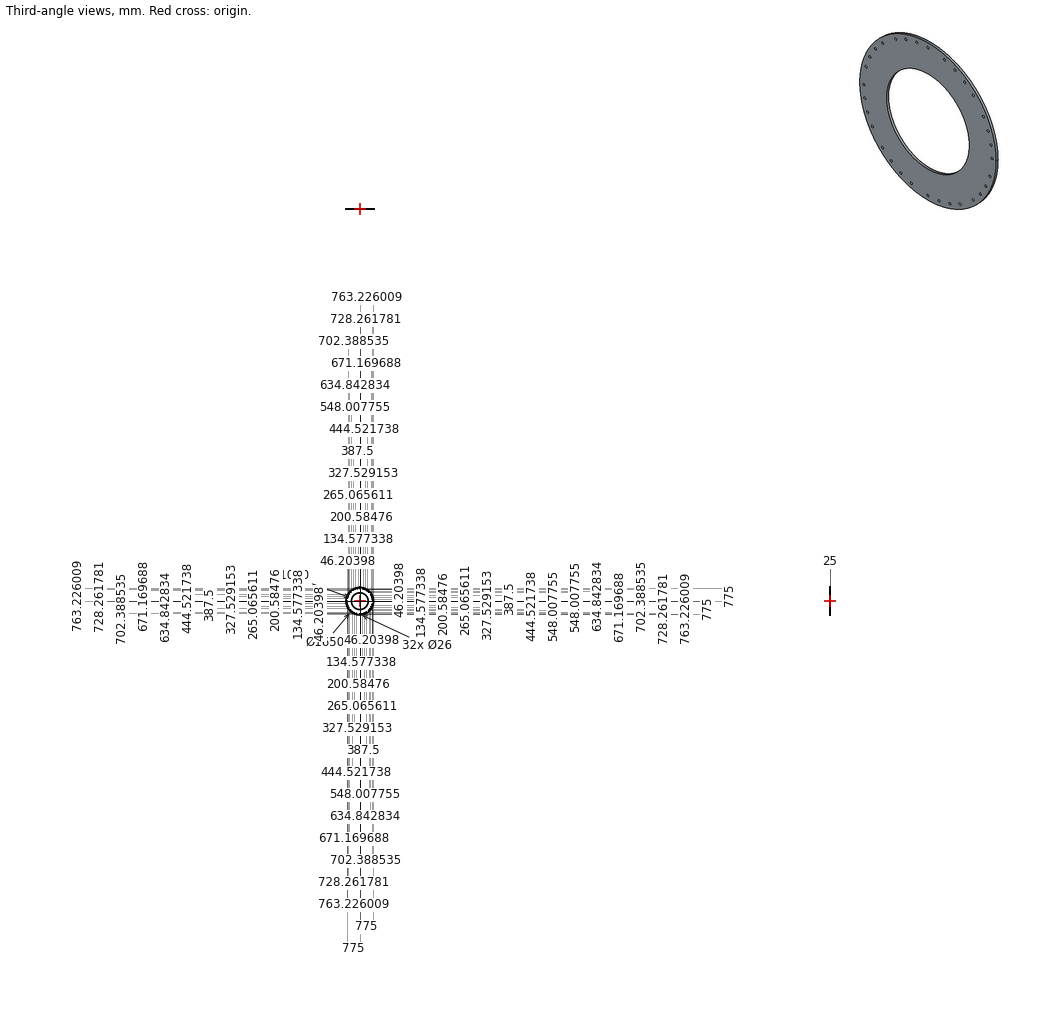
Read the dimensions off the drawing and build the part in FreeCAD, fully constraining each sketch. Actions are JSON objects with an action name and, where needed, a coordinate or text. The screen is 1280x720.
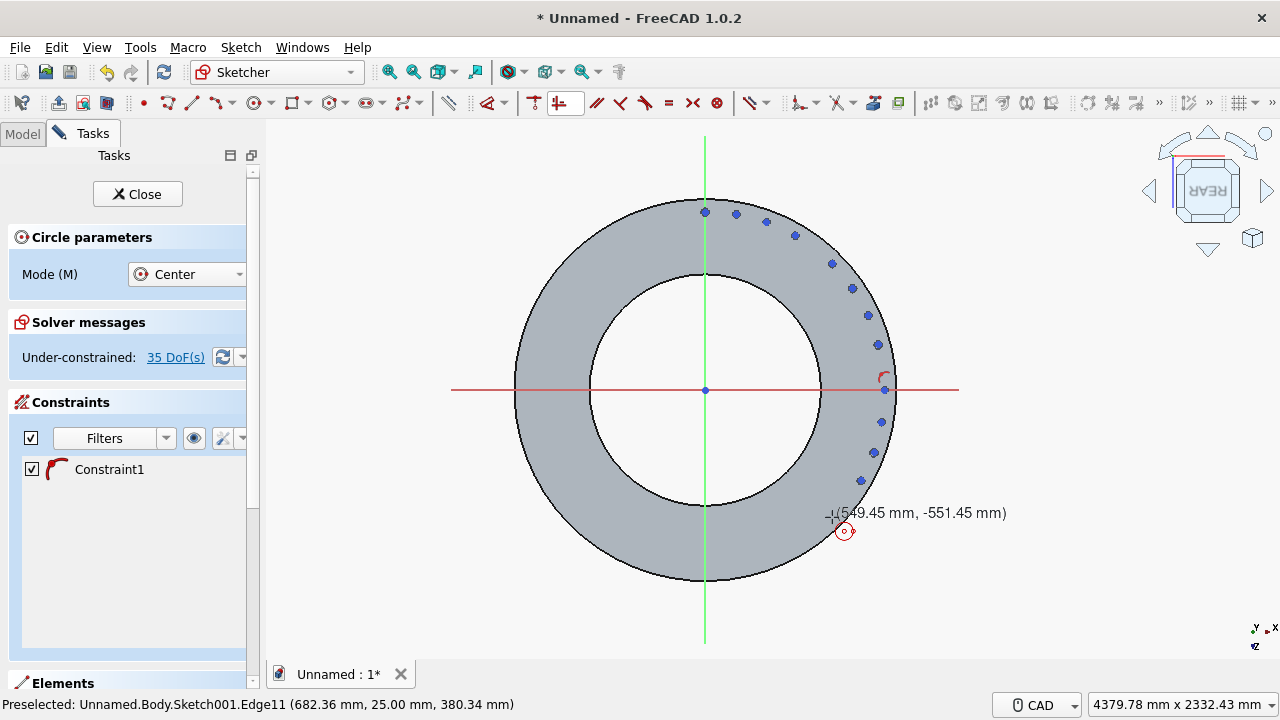
{"action": "left_click", "coordinate": [832, 517]}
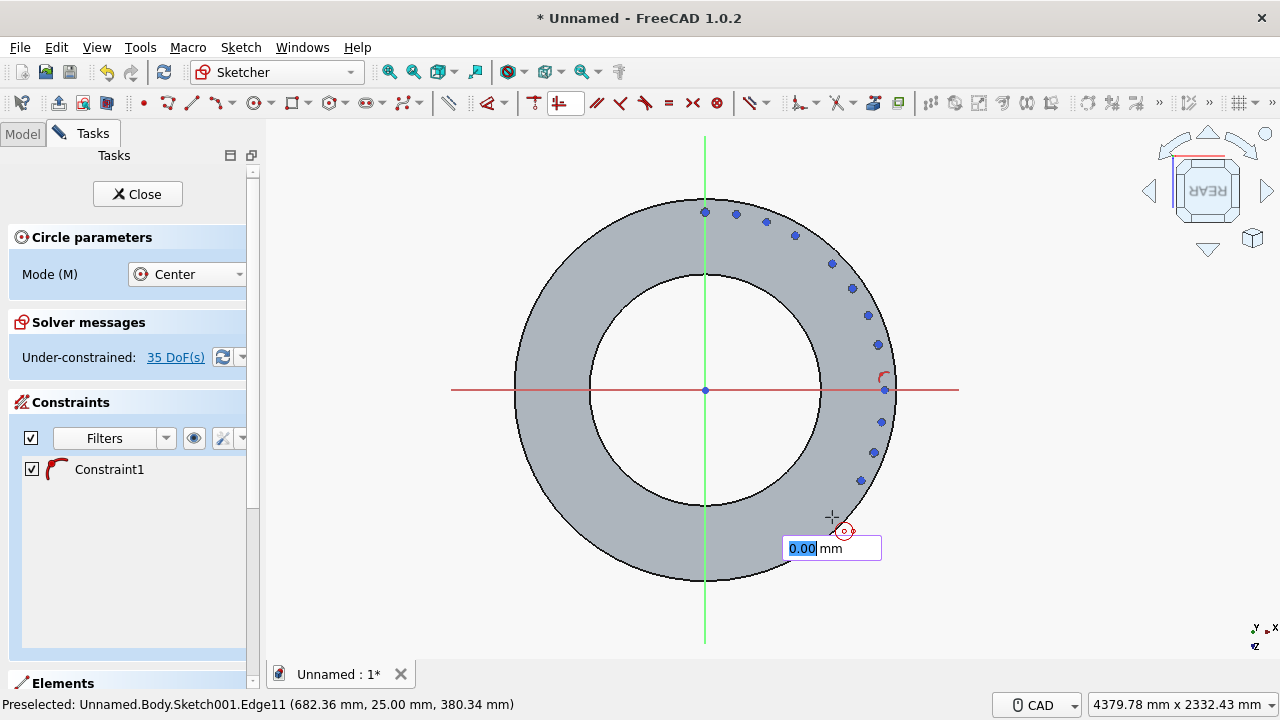
{"action": "scroll", "coordinate": [834, 515], "scroll_direction": "up", "scroll_amount": 9}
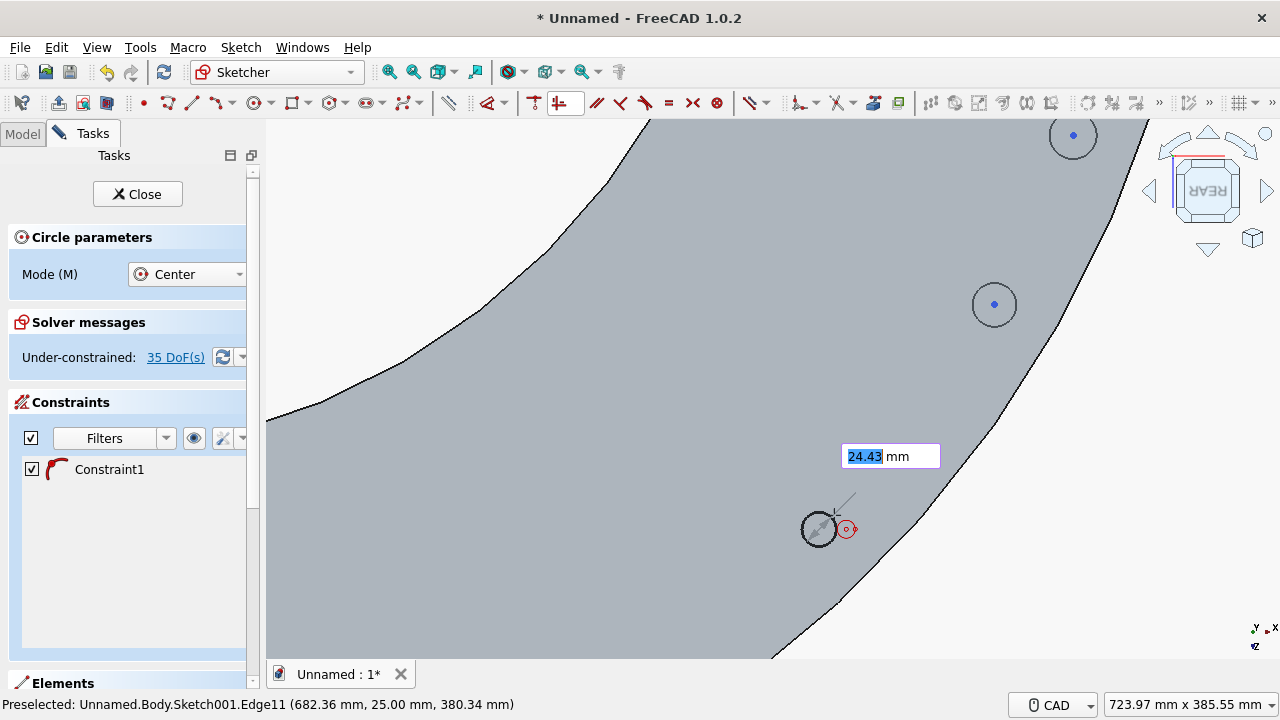
{"action": "left_click", "coordinate": [833, 510]}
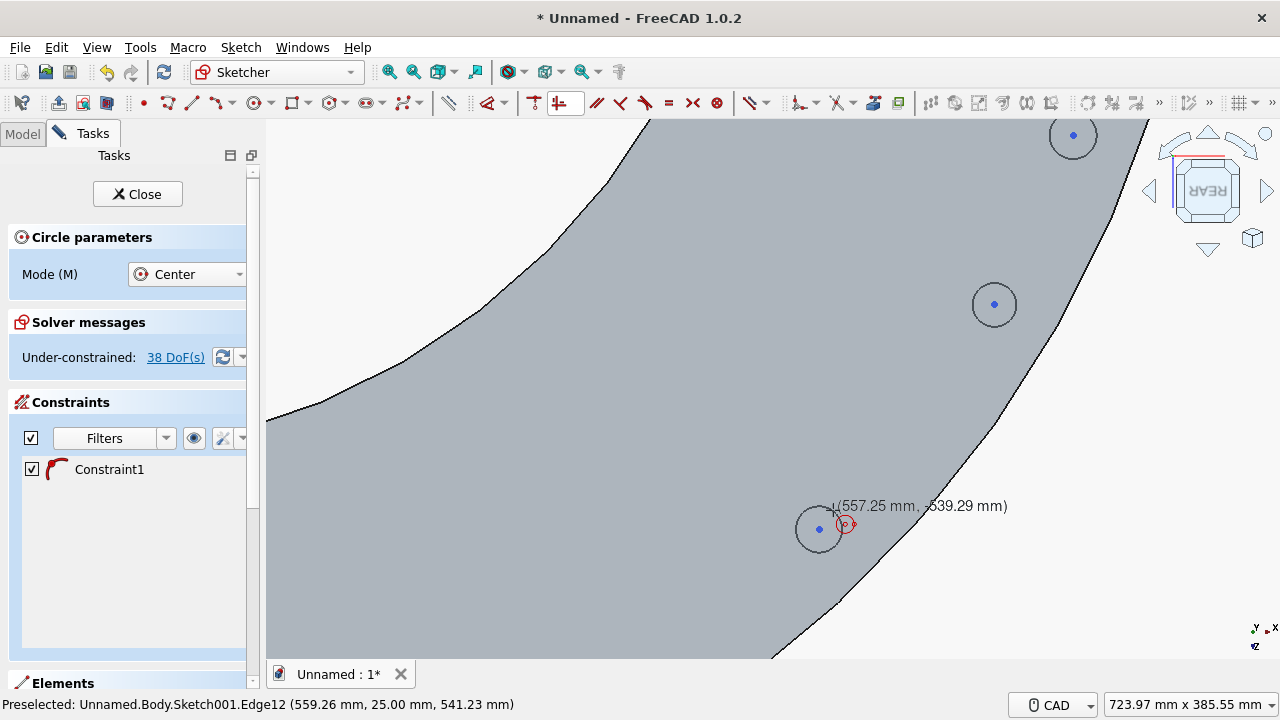
{"action": "scroll", "coordinate": [834, 514], "scroll_direction": "down", "scroll_amount": 9}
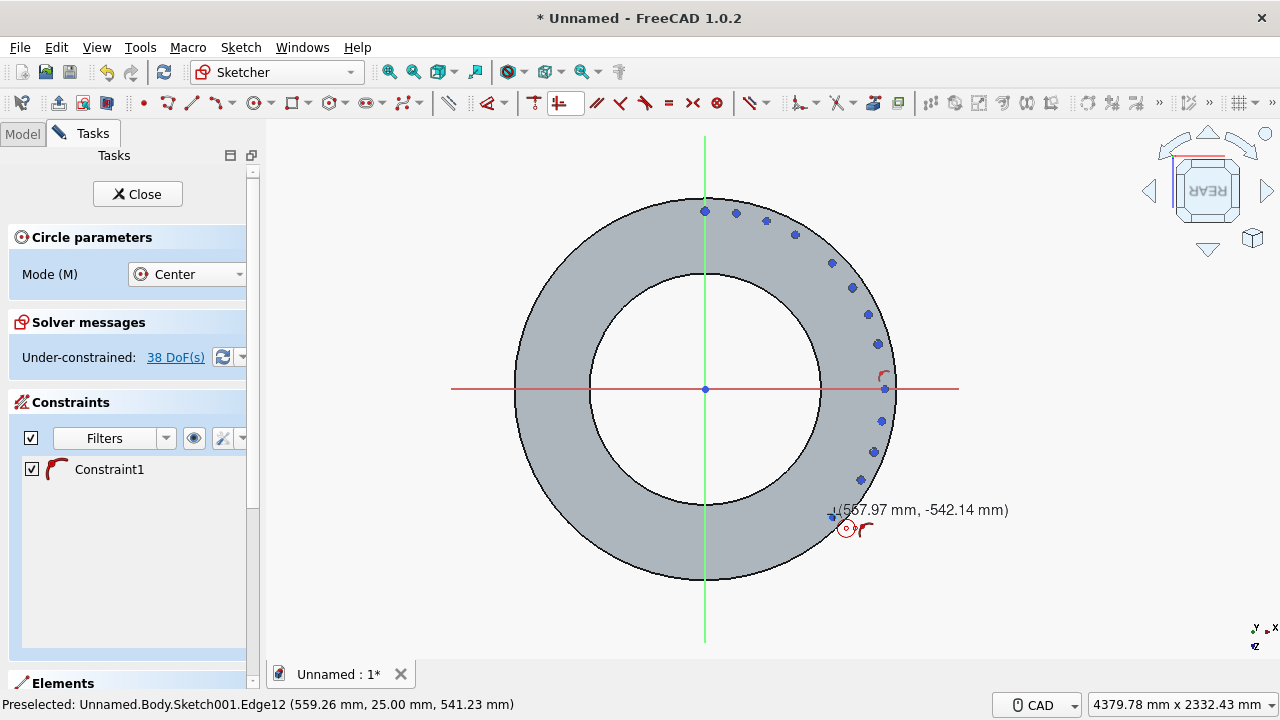
{"action": "scroll", "coordinate": [808, 536], "scroll_direction": "up", "scroll_amount": 11}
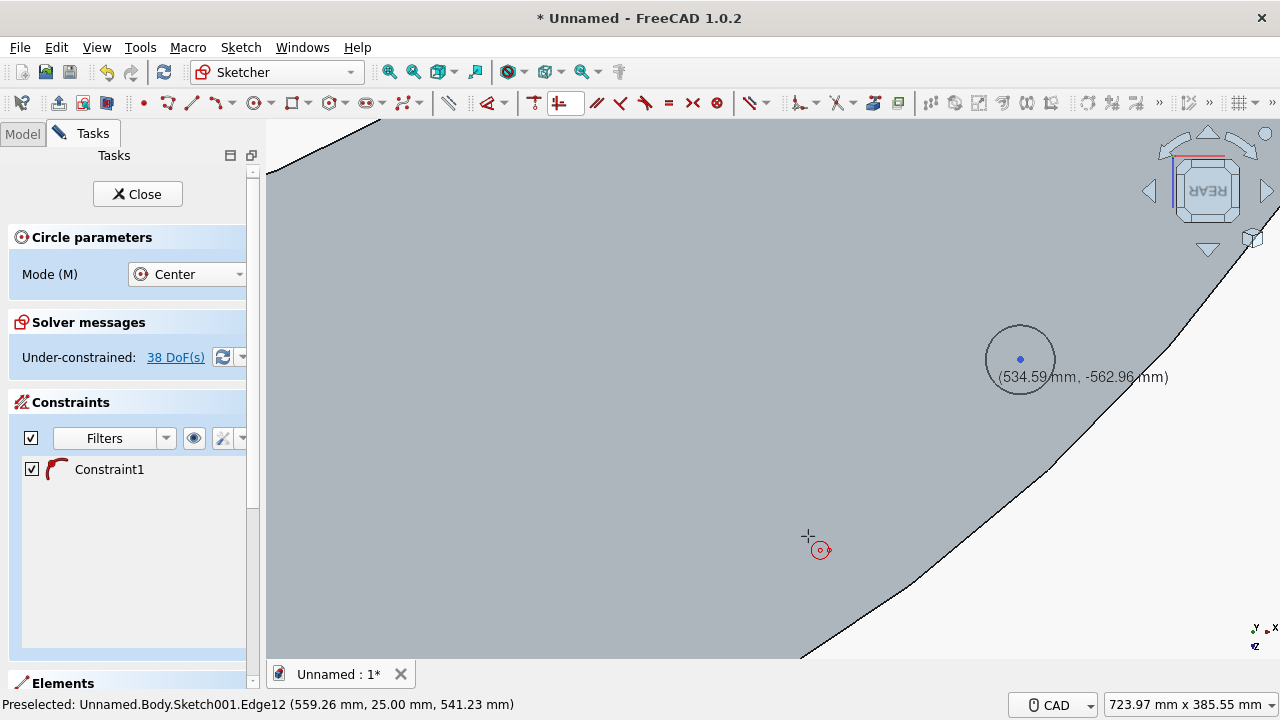
{"action": "scroll", "coordinate": [808, 536], "scroll_direction": "down", "scroll_amount": 11}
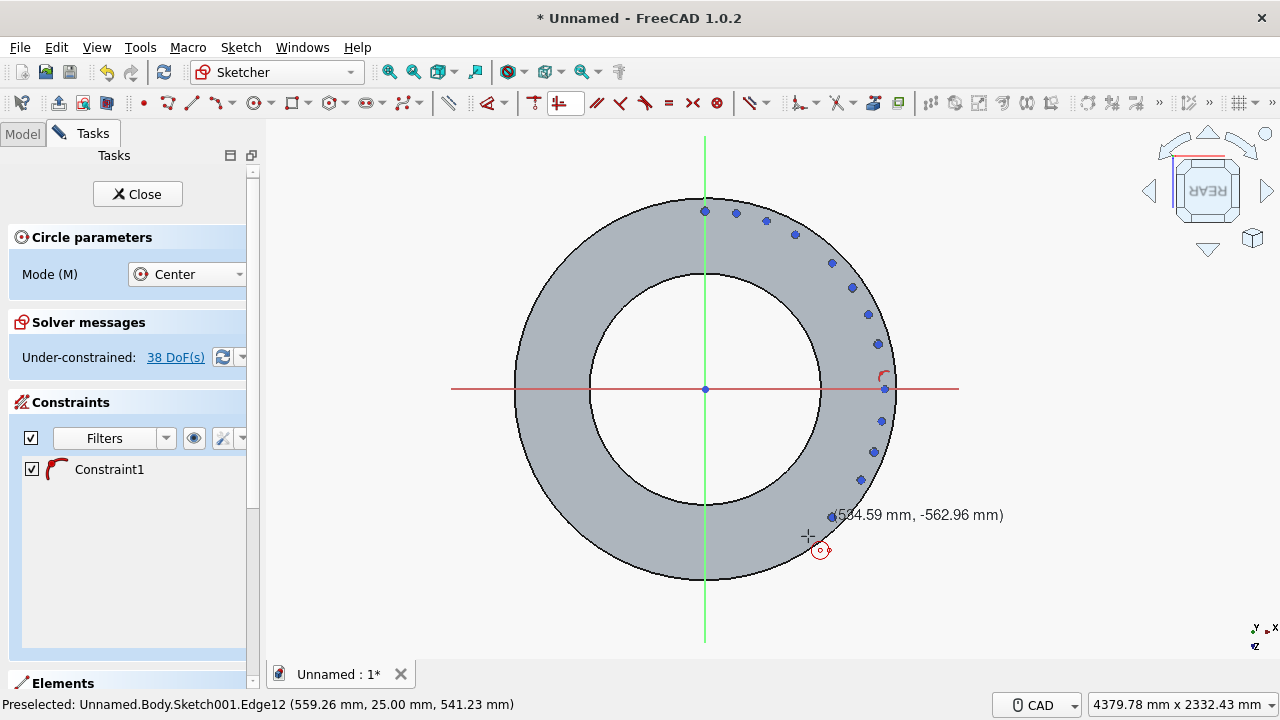
{"action": "left_click", "coordinate": [808, 536]}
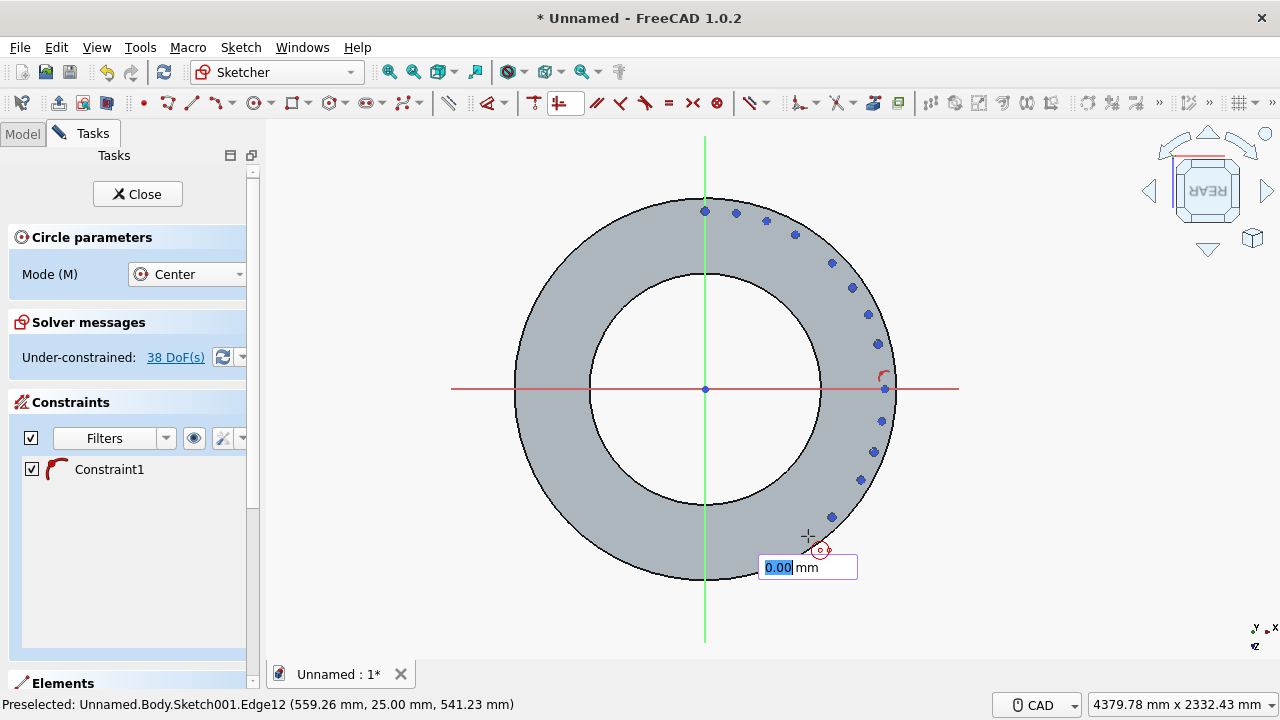
{"action": "scroll", "coordinate": [810, 534], "scroll_direction": "up", "scroll_amount": 9}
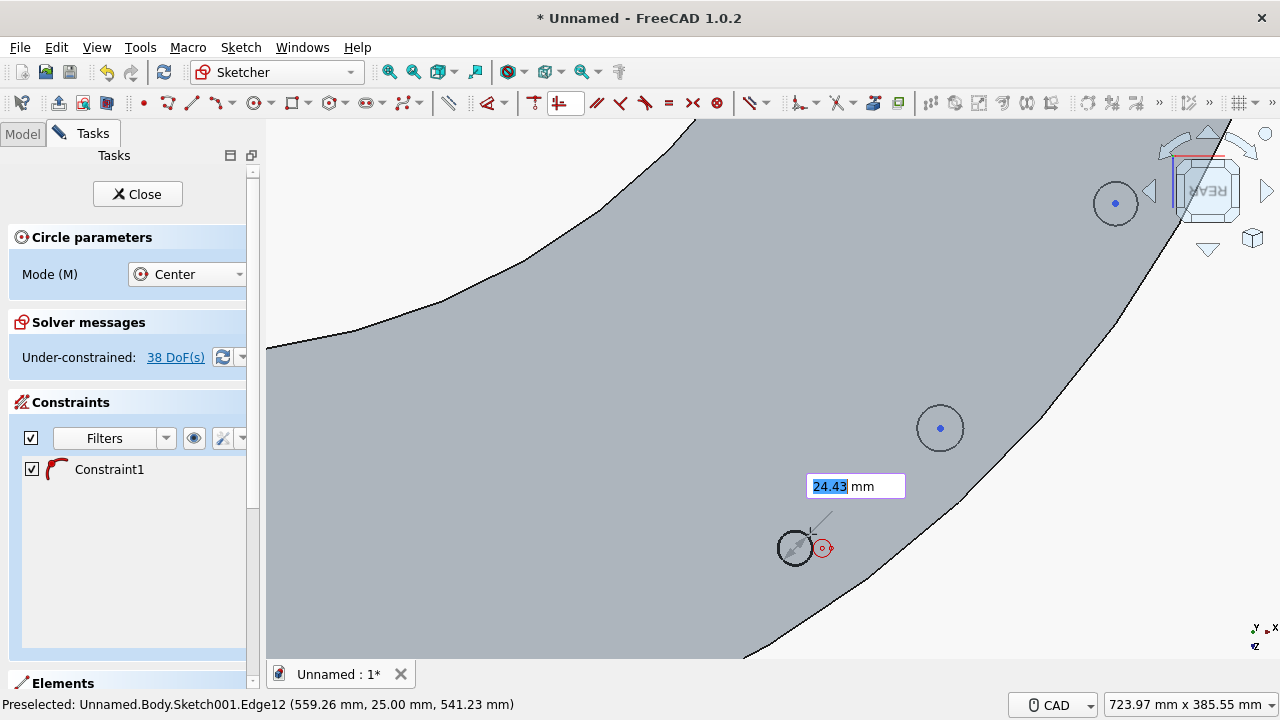
{"action": "left_click", "coordinate": [809, 531]}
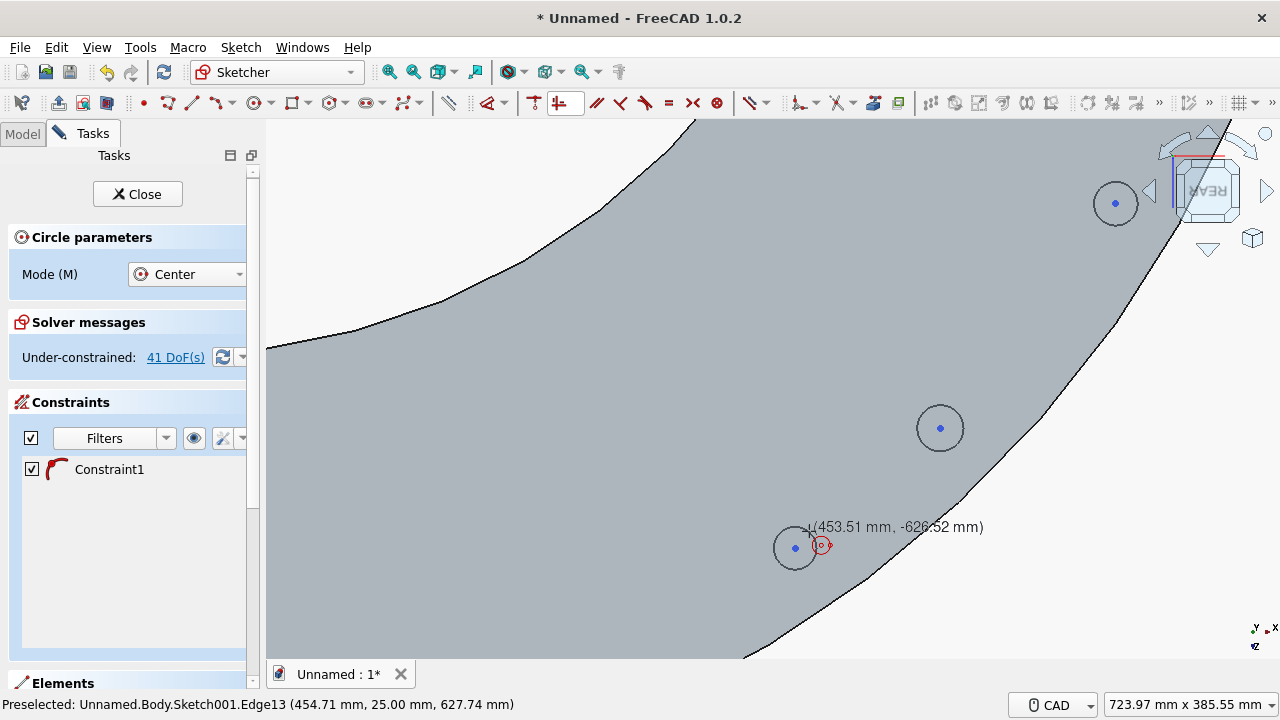
{"action": "scroll", "coordinate": [810, 534], "scroll_direction": "down", "scroll_amount": 9}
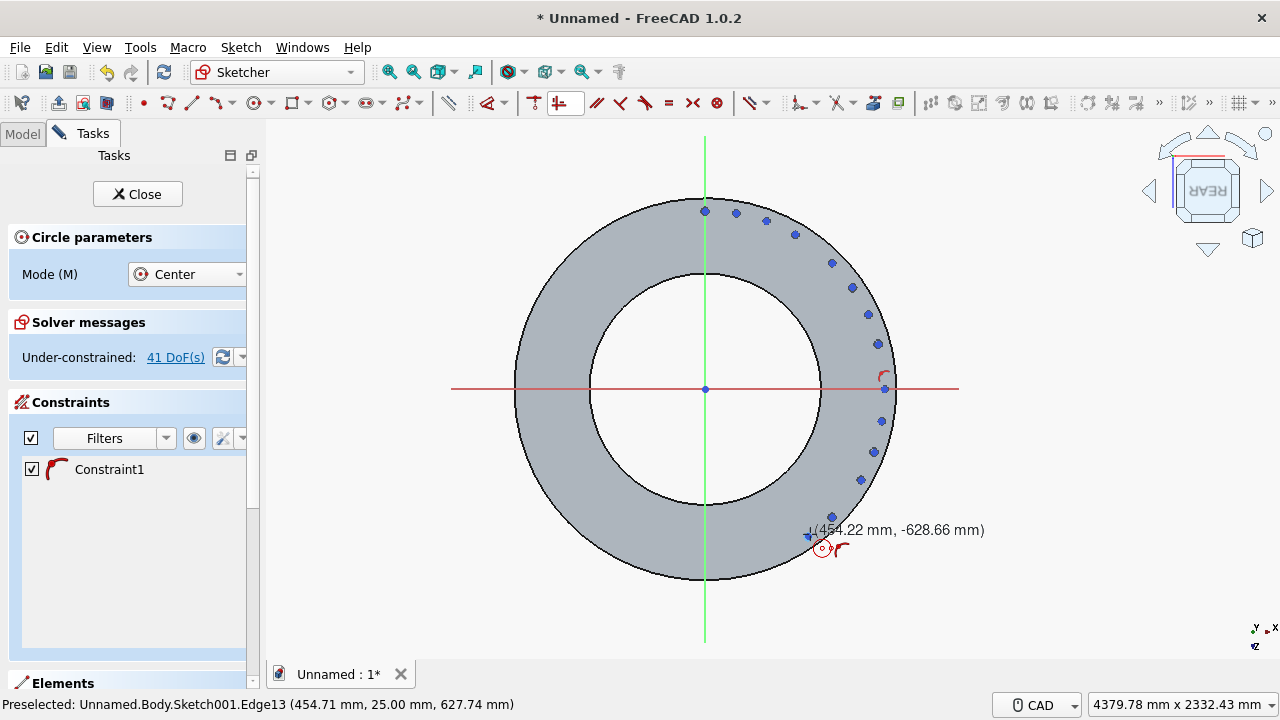
{"action": "scroll", "coordinate": [781, 552], "scroll_direction": "up", "scroll_amount": 11}